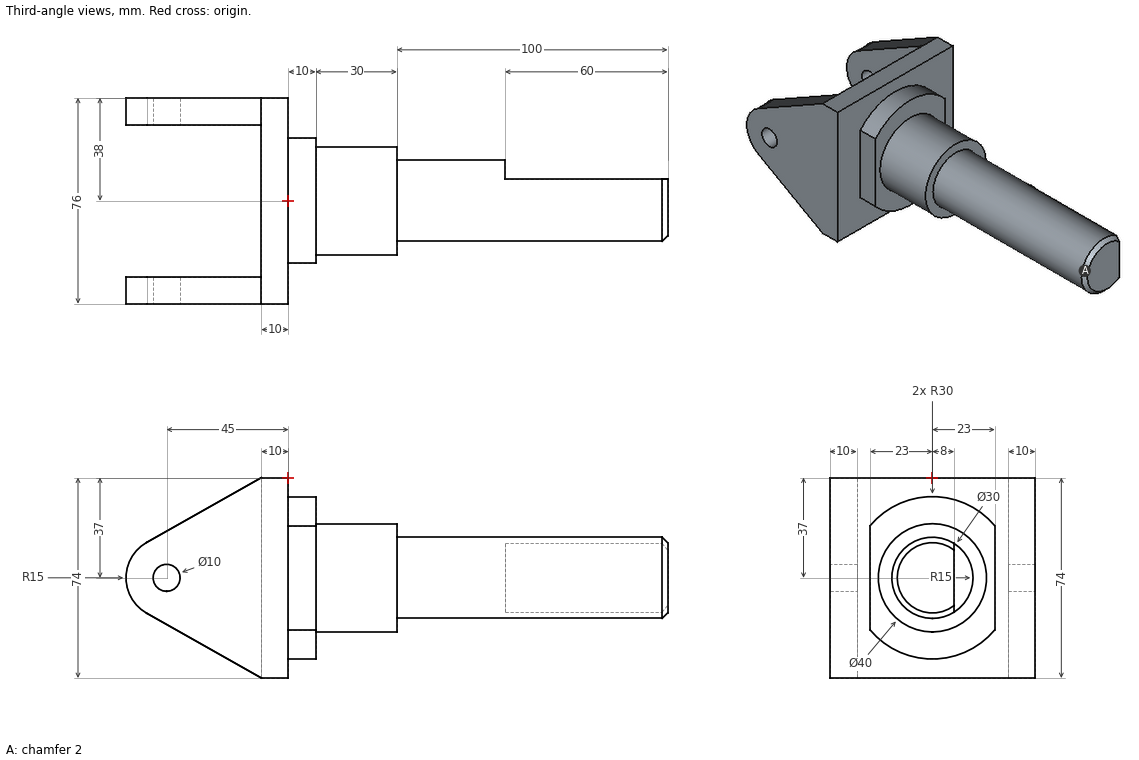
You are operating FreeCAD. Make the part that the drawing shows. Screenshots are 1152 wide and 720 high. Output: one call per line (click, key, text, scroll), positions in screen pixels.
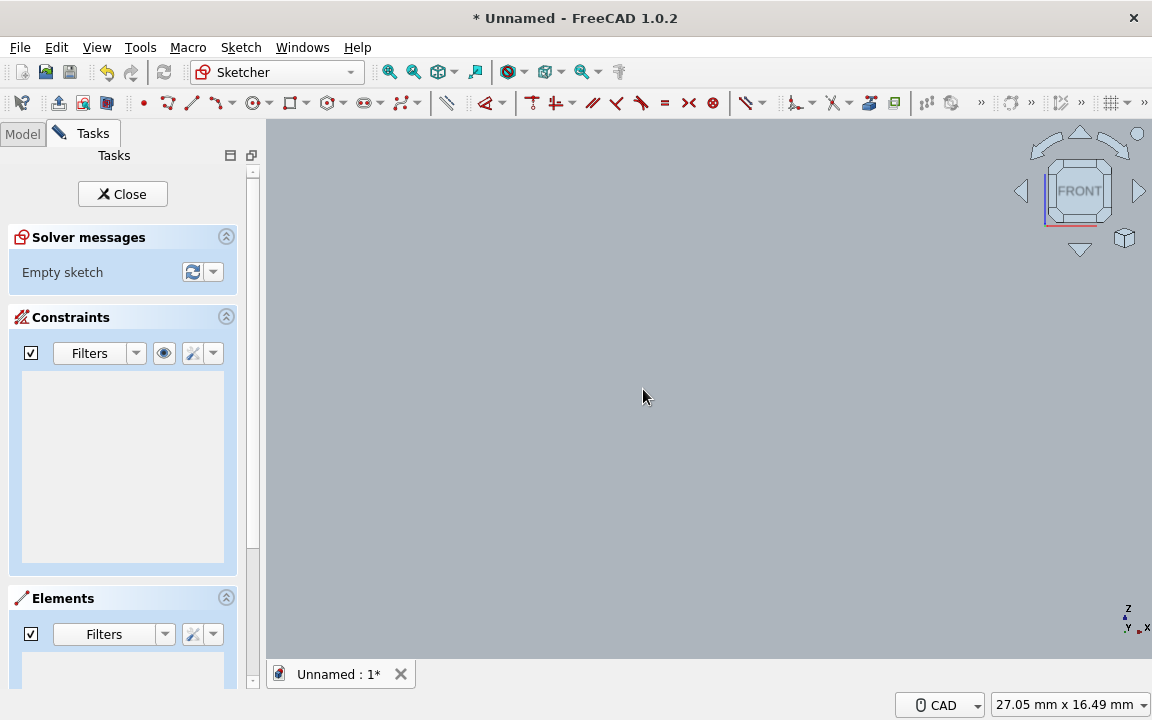
click(254, 104)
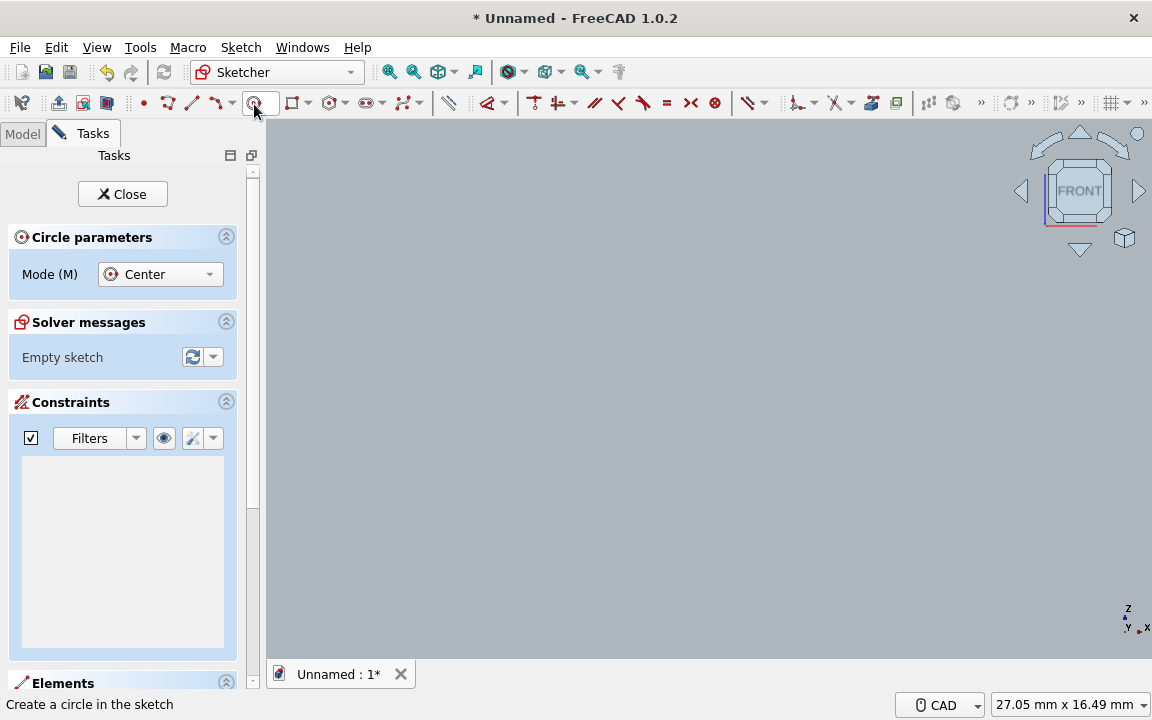
click(636, 386)
click(751, 270)
key(Escape)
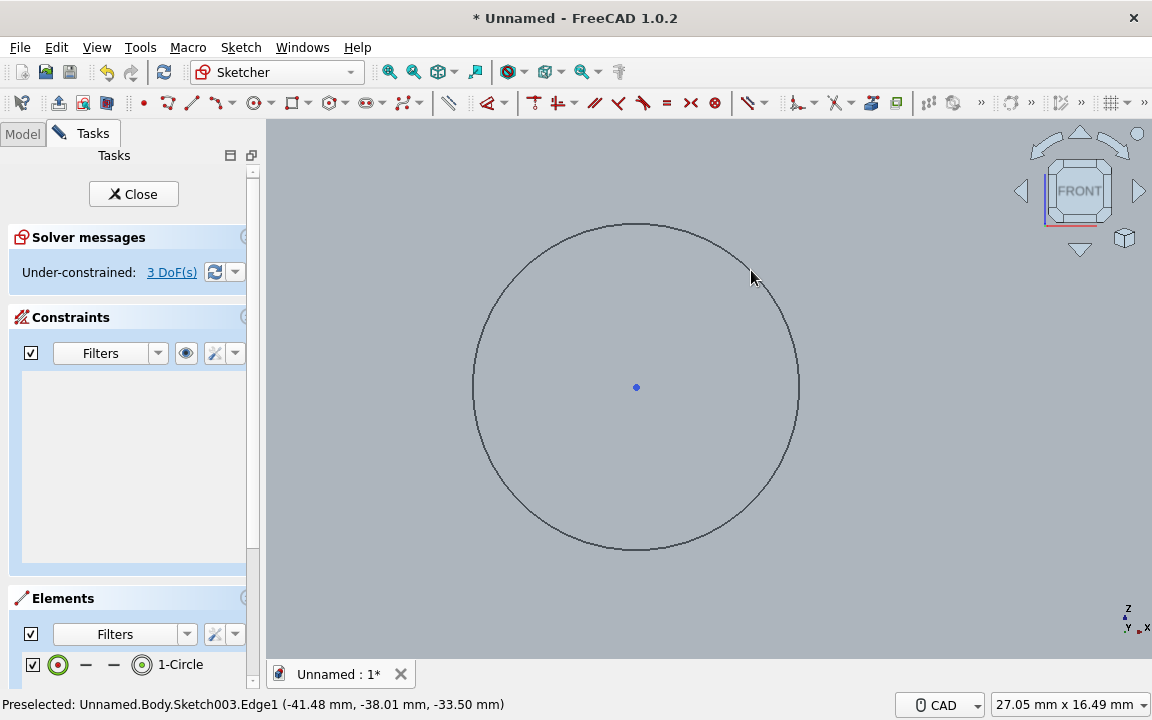
click(488, 104)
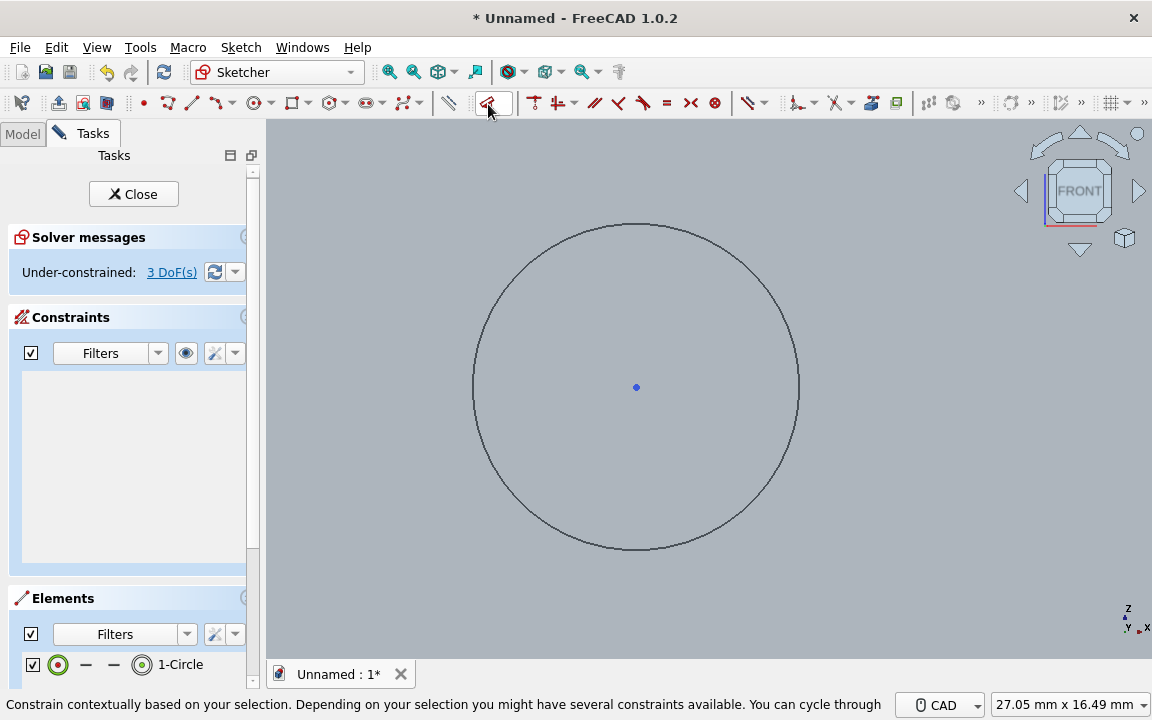
click(751, 271)
click(774, 248)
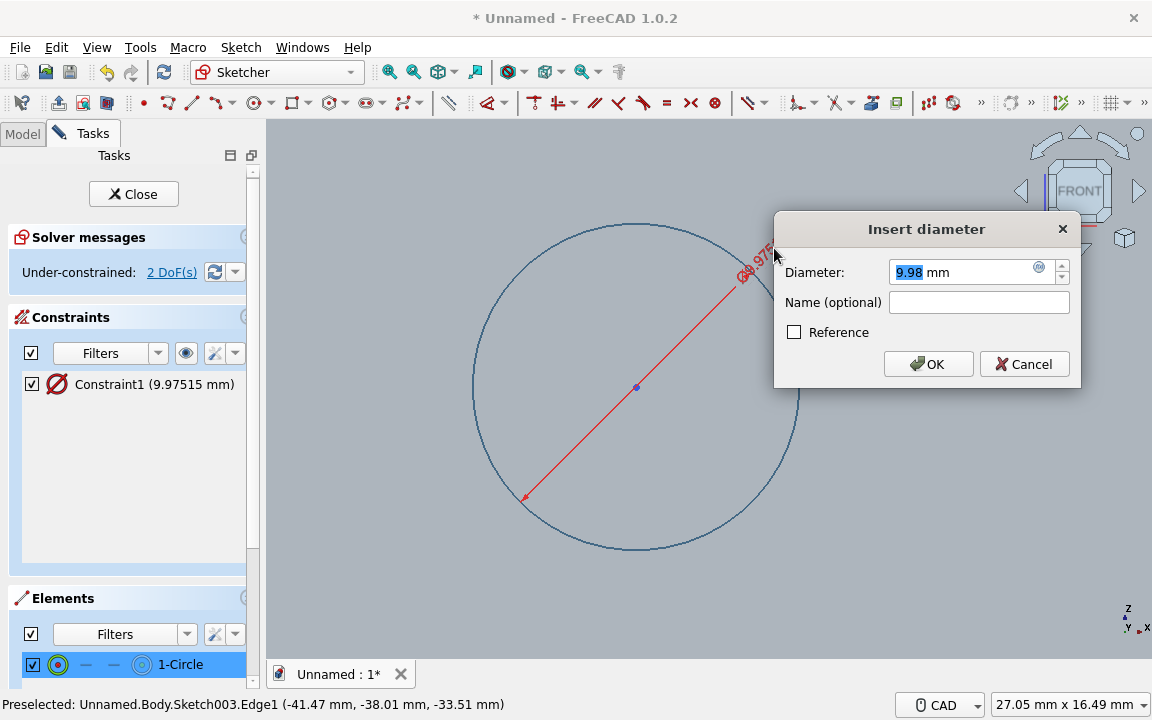
text(10)
key(Return)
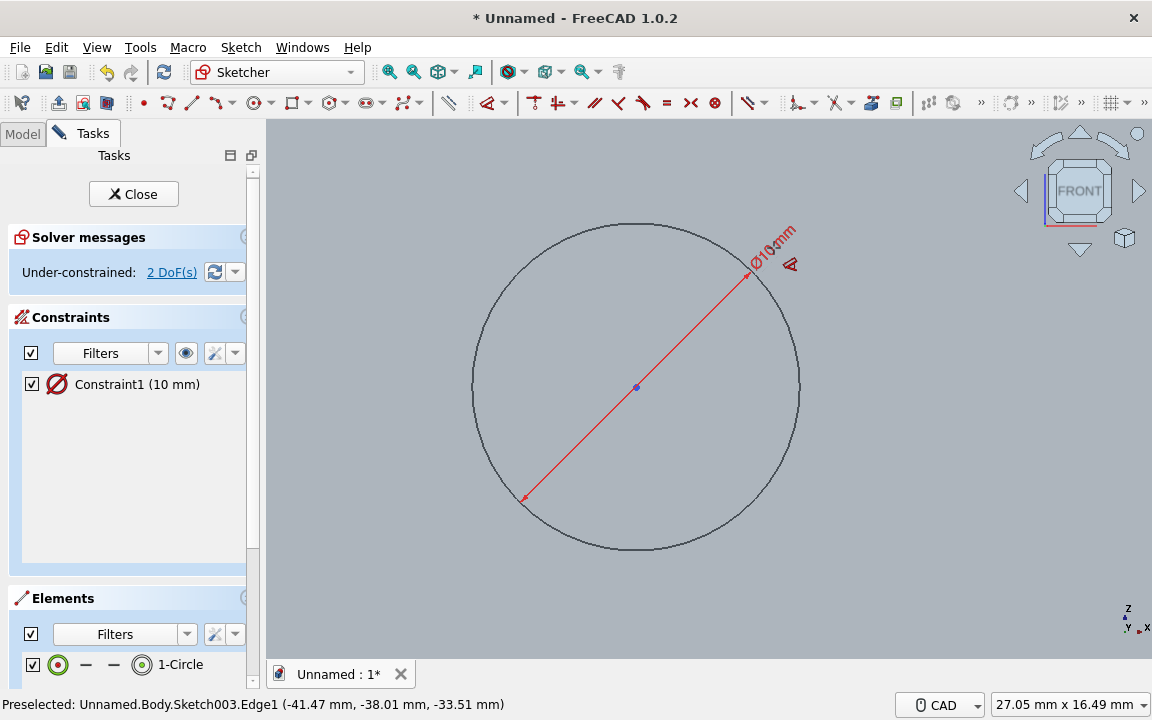
click(636, 387)
click(811, 421)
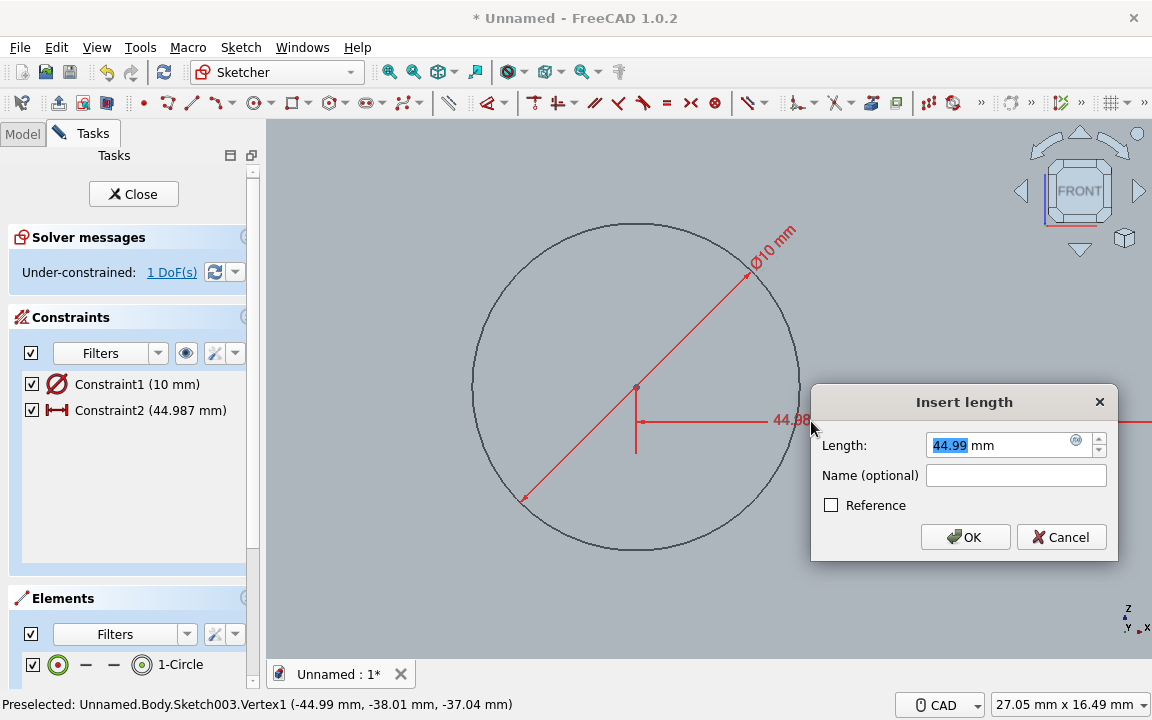
text(45)
key(Return)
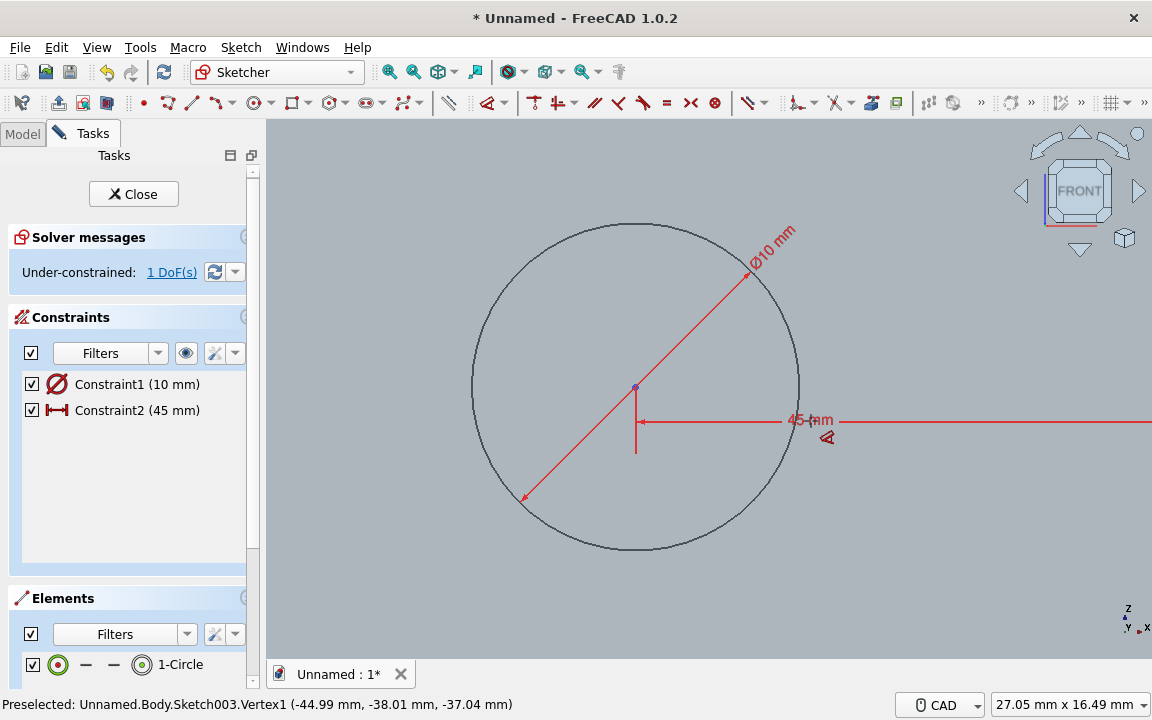
click(636, 387)
click(602, 267)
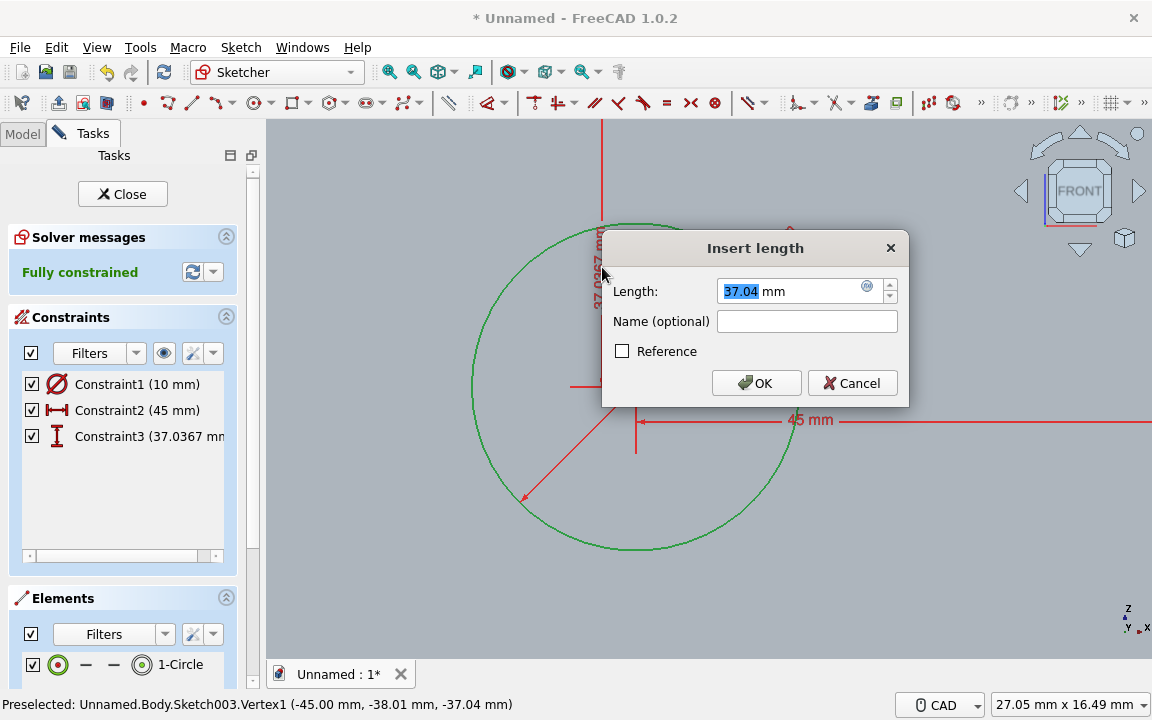
text(37)
key(Return)
key(Escape)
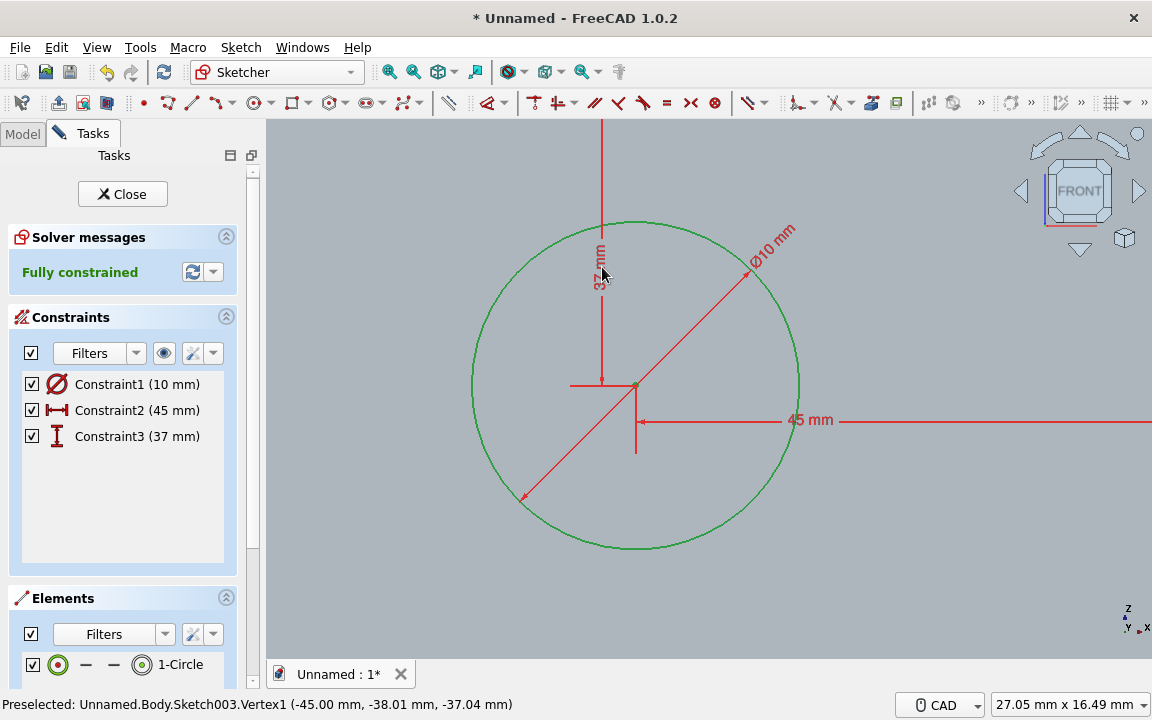
click(123, 194)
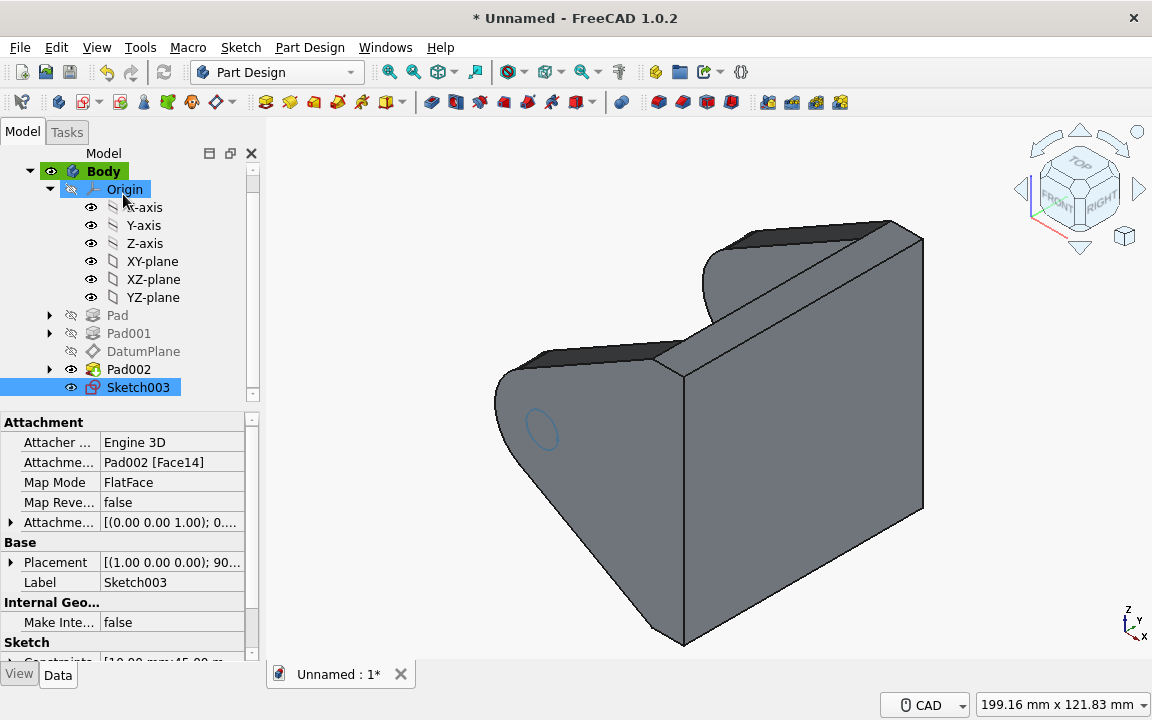
click(432, 102)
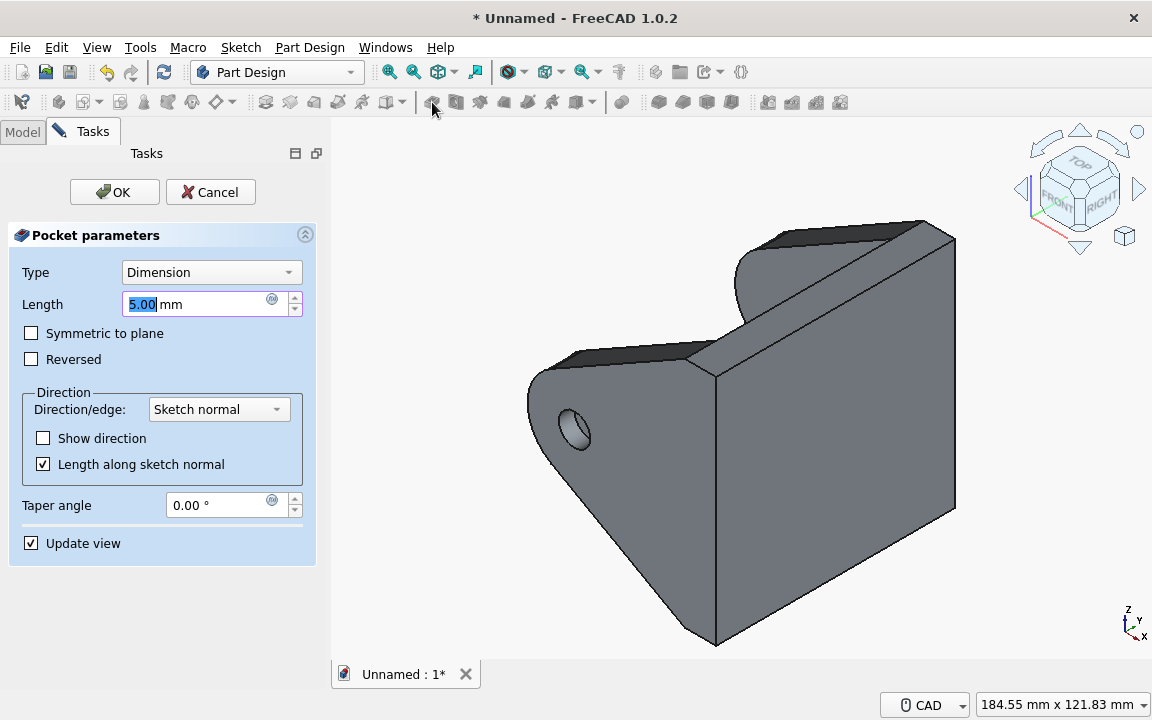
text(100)
key(Tab)